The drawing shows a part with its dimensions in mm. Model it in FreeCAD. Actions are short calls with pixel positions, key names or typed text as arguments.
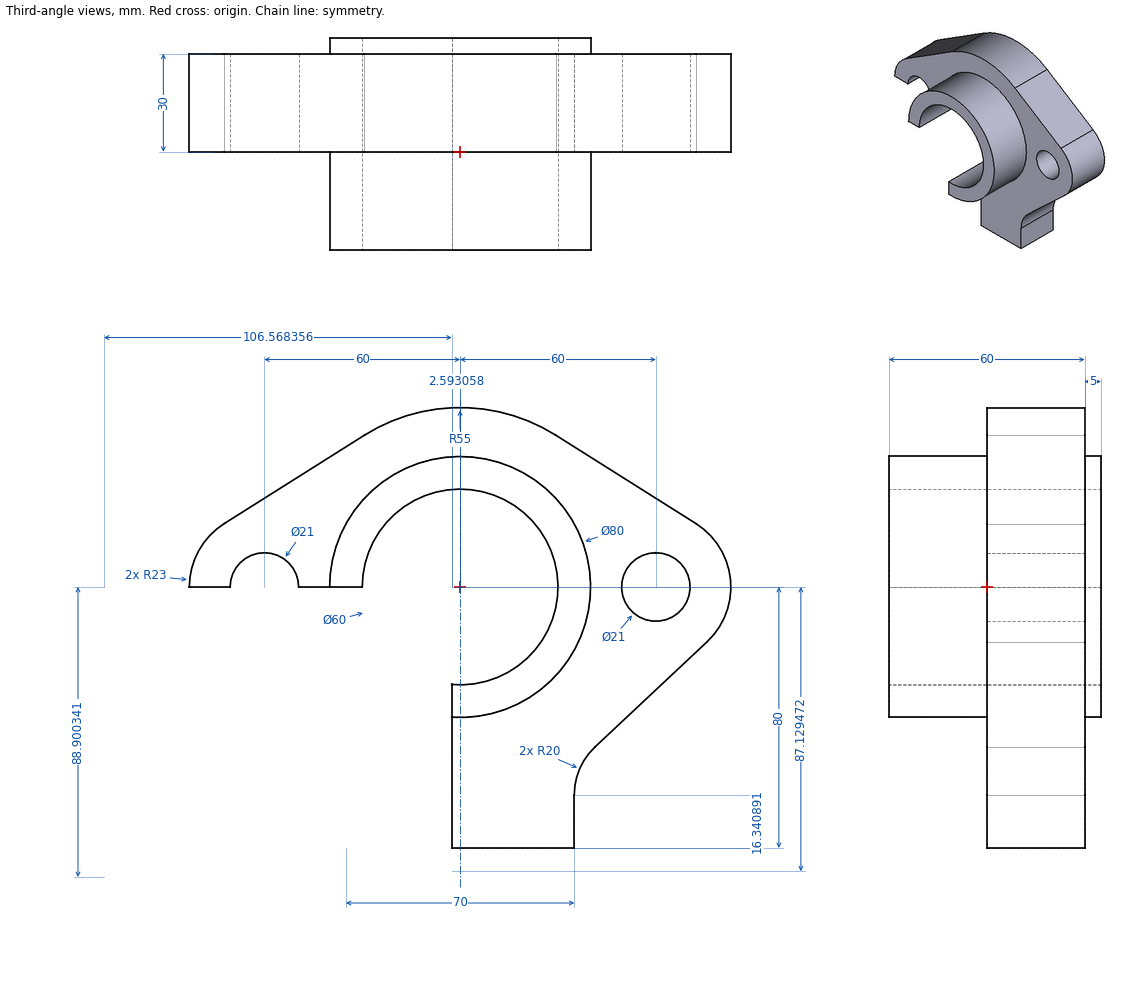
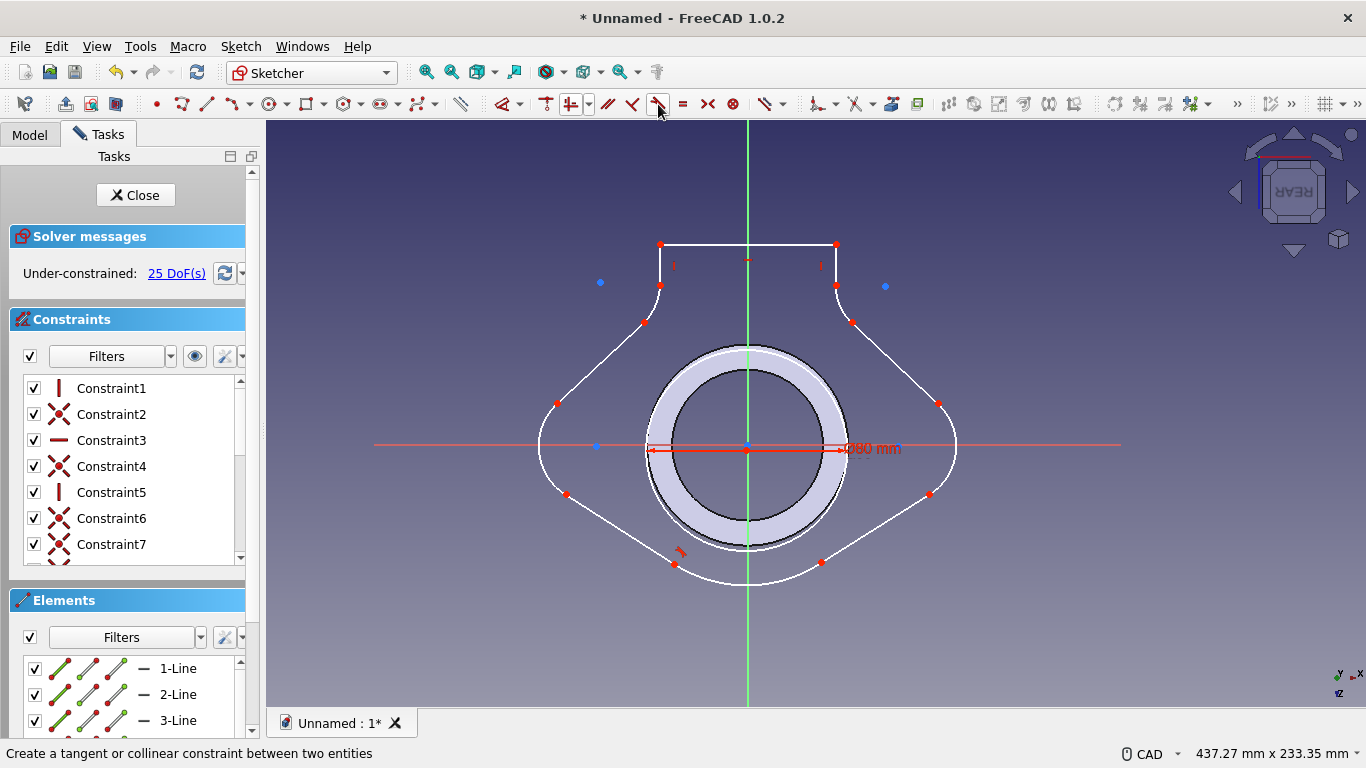
click(598, 516)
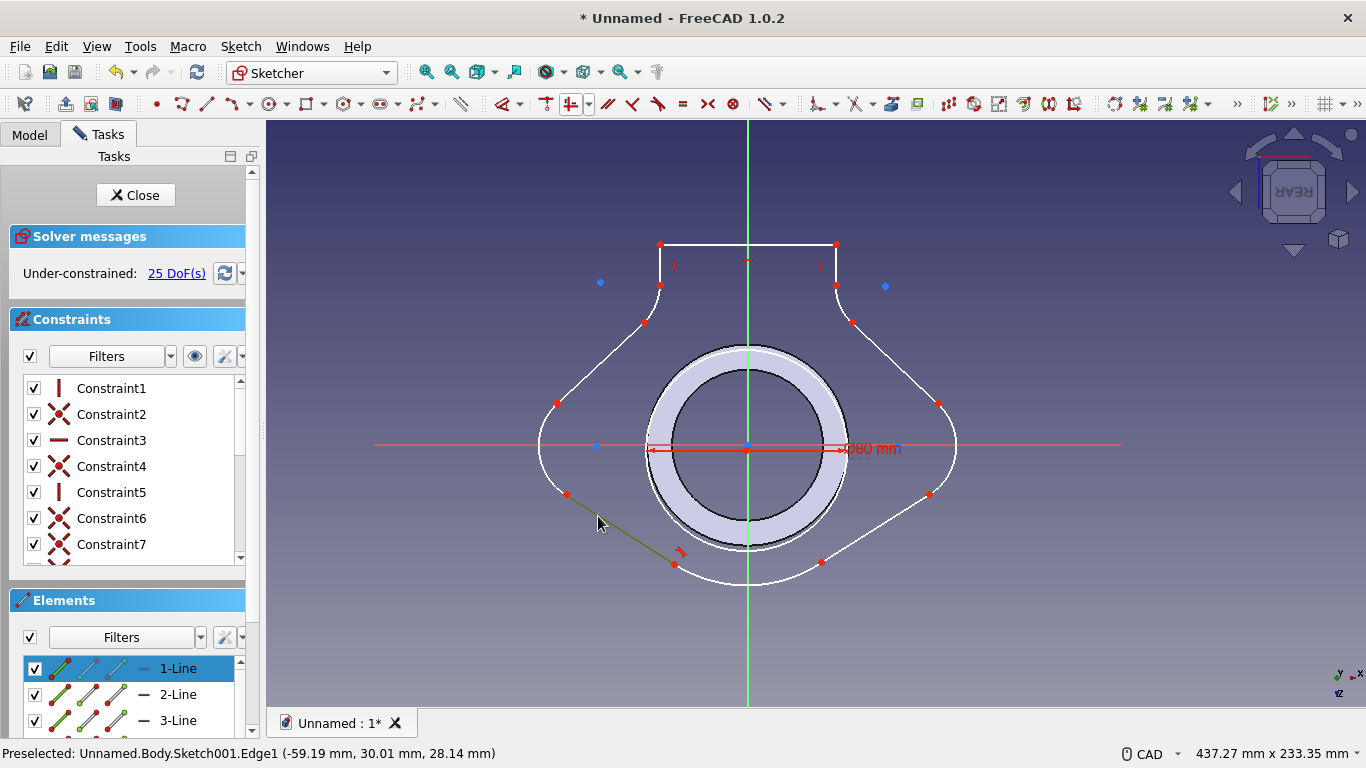
click(541, 431)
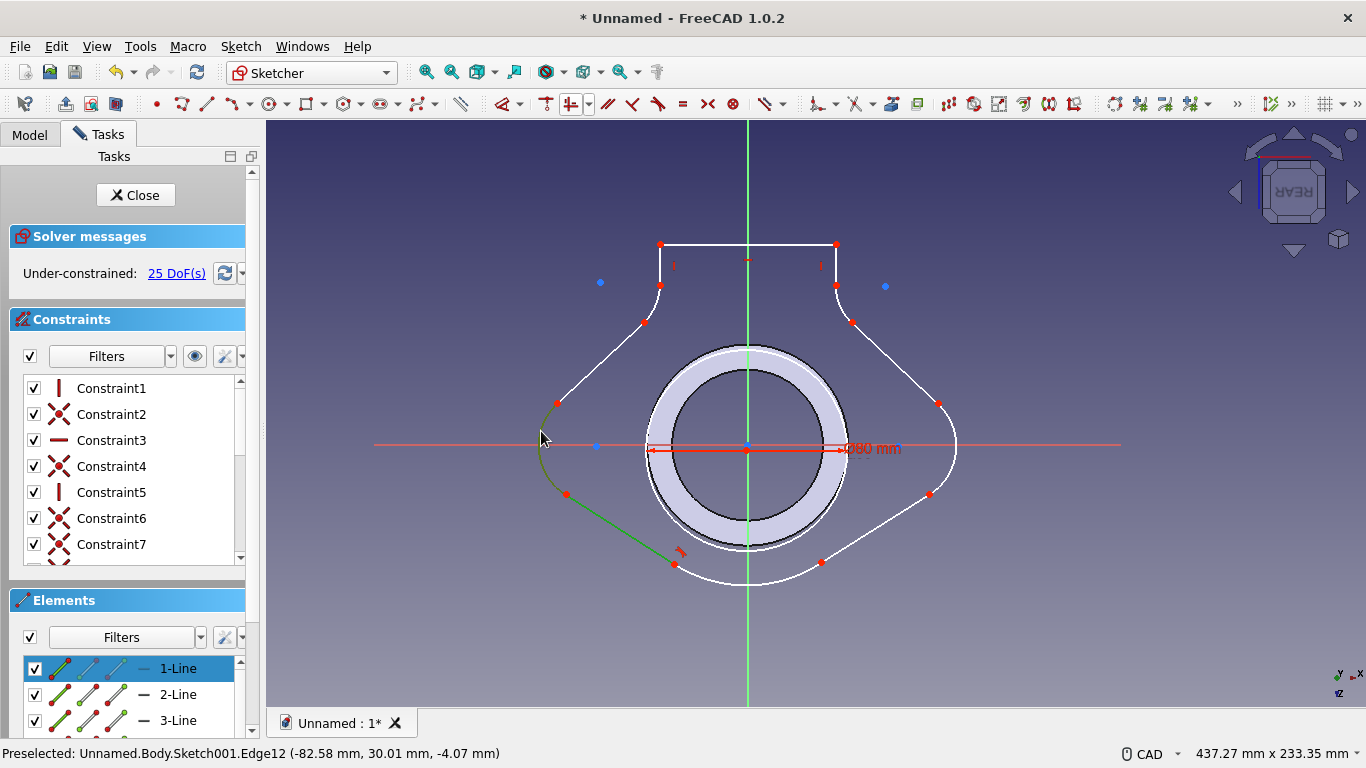
click(658, 104)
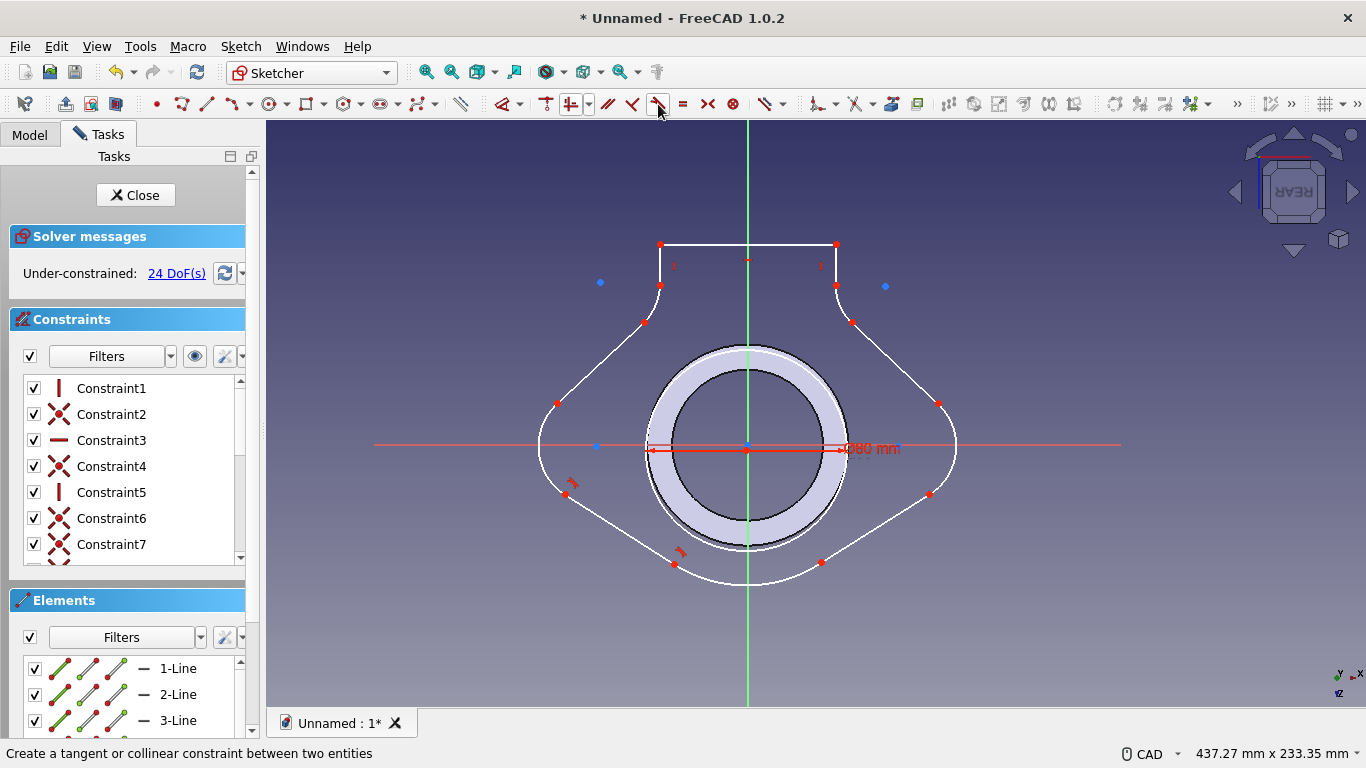
click(853, 543)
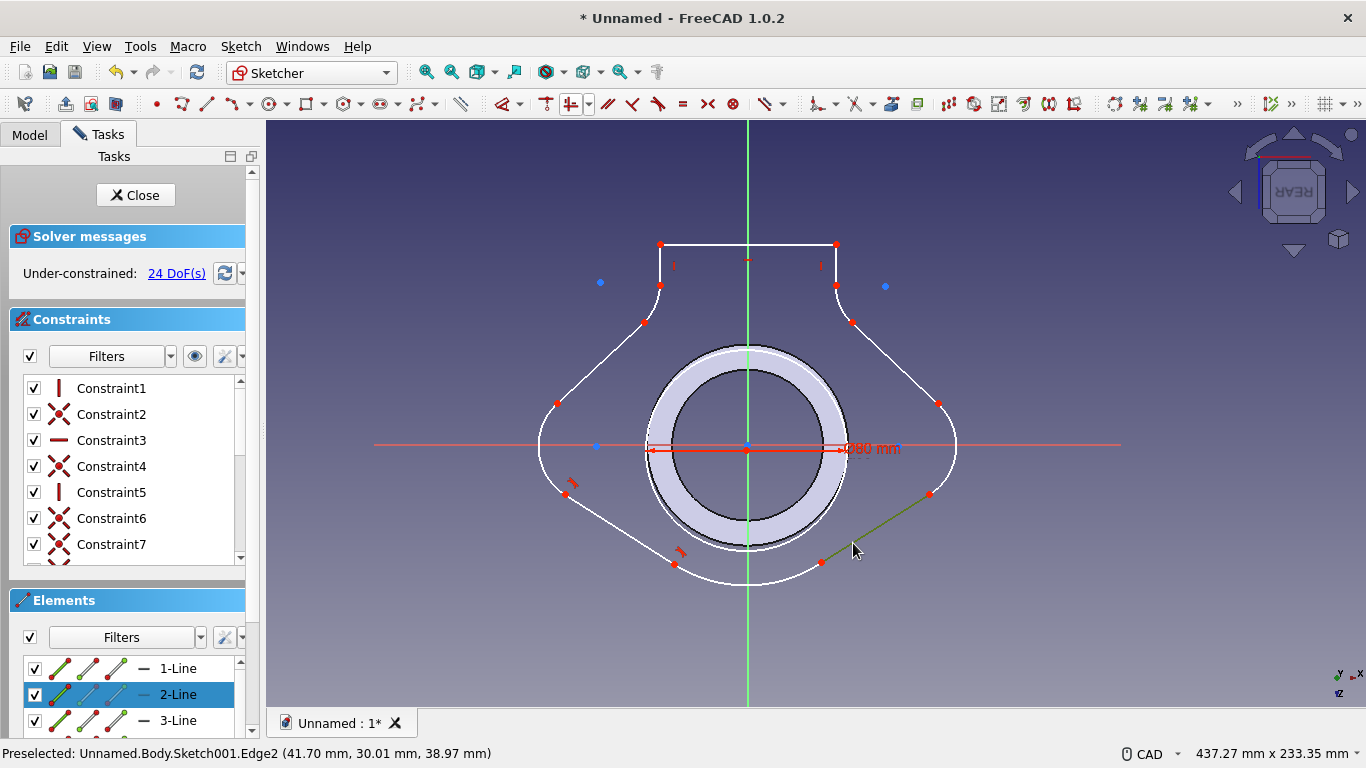
click(717, 582)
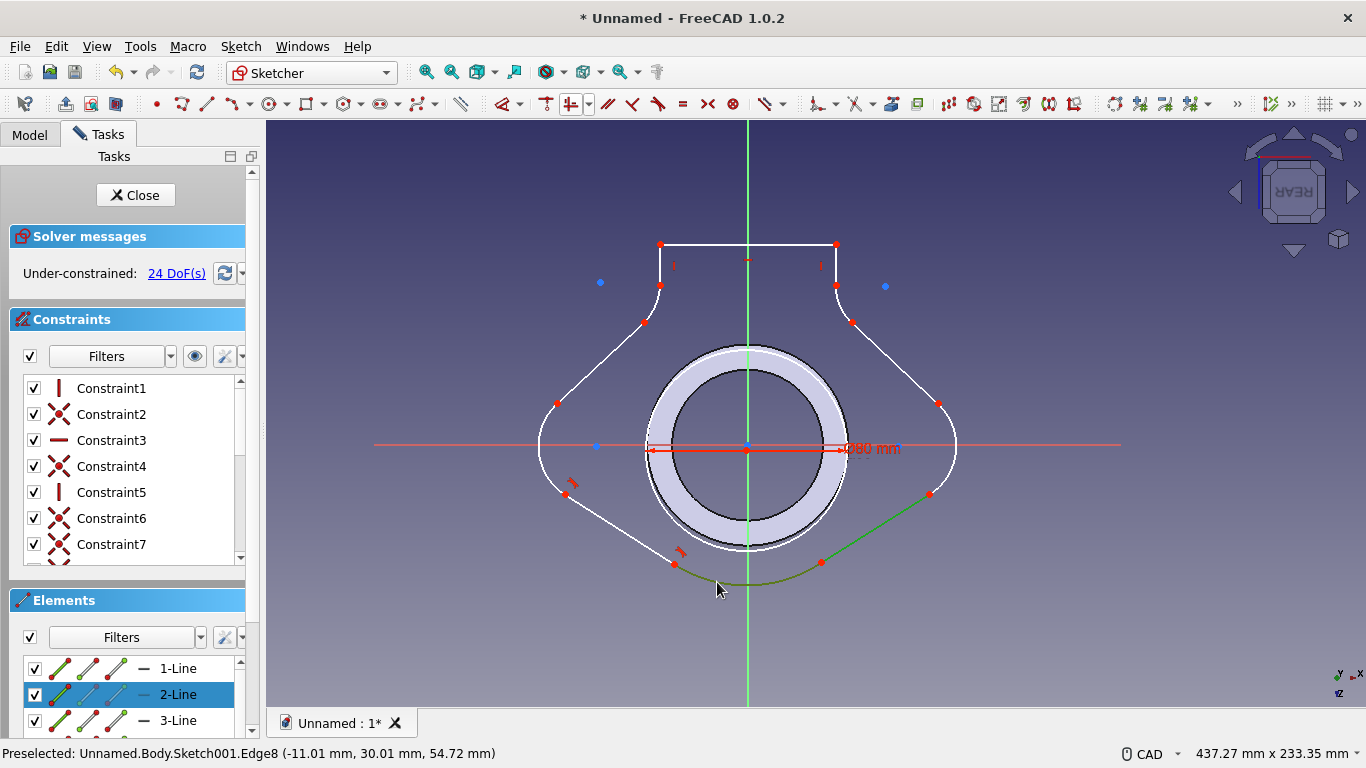
click(658, 104)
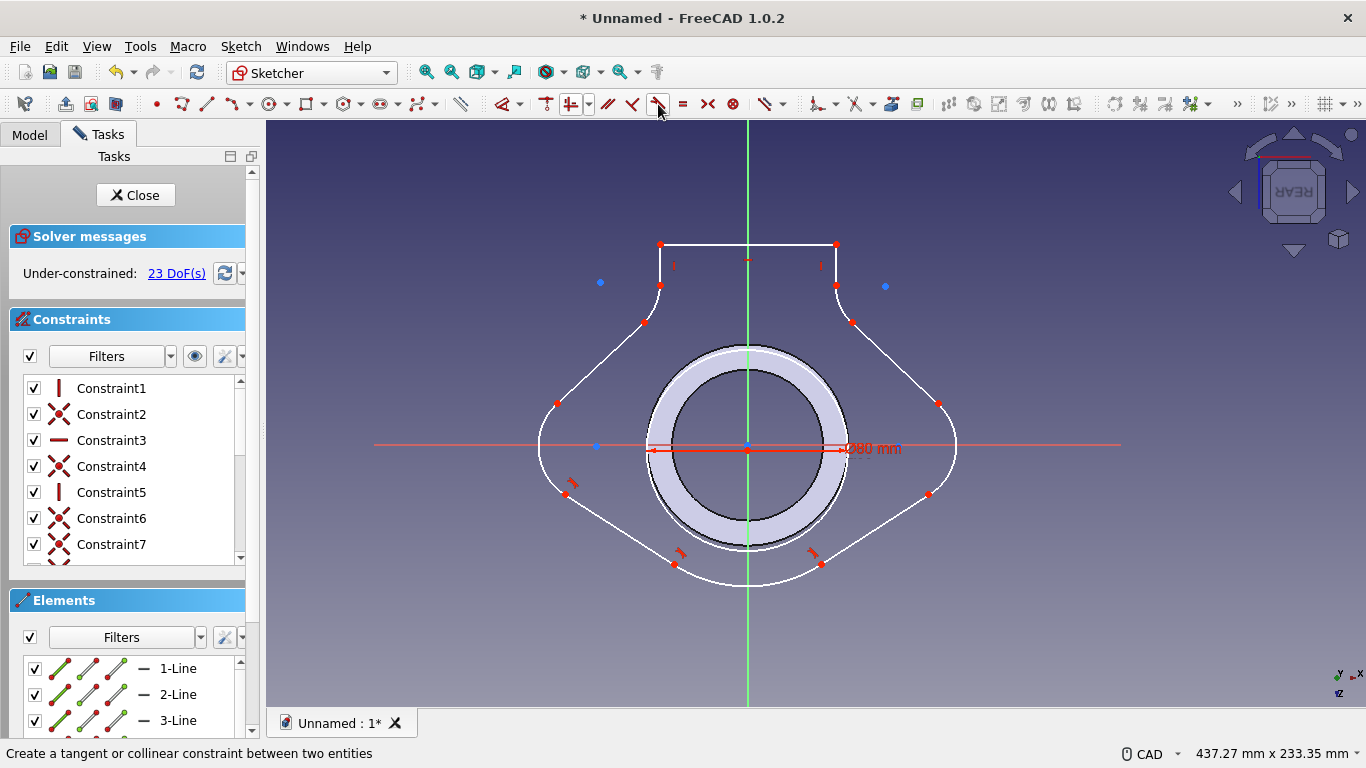
click(853, 544)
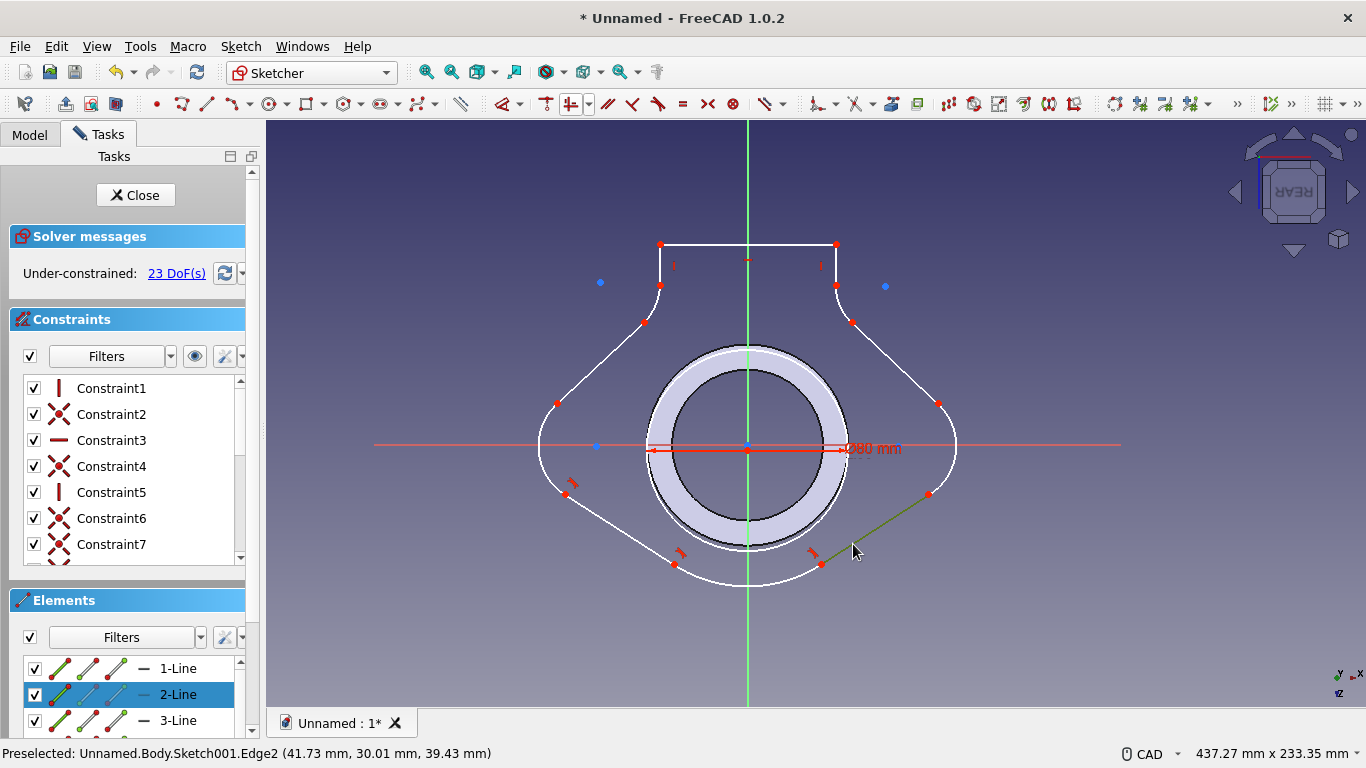
click(950, 472)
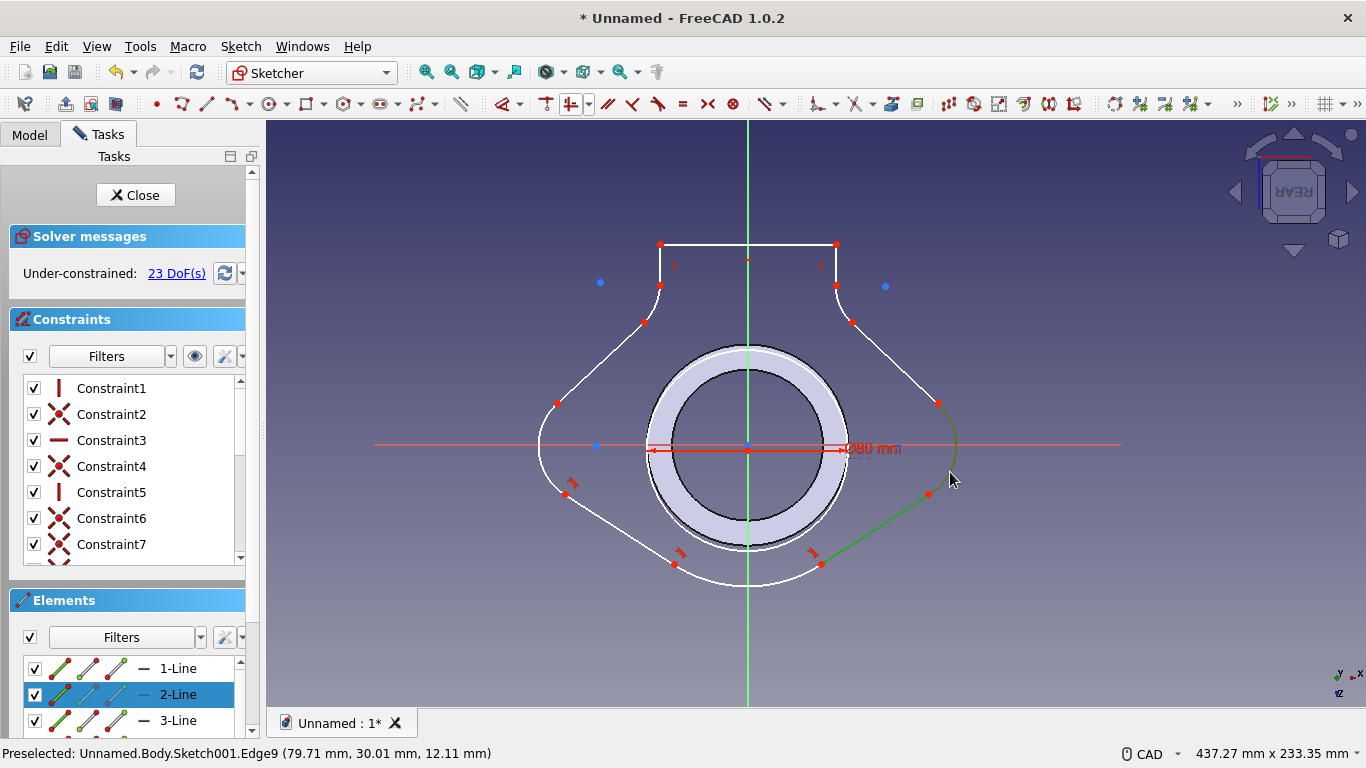
click(658, 104)